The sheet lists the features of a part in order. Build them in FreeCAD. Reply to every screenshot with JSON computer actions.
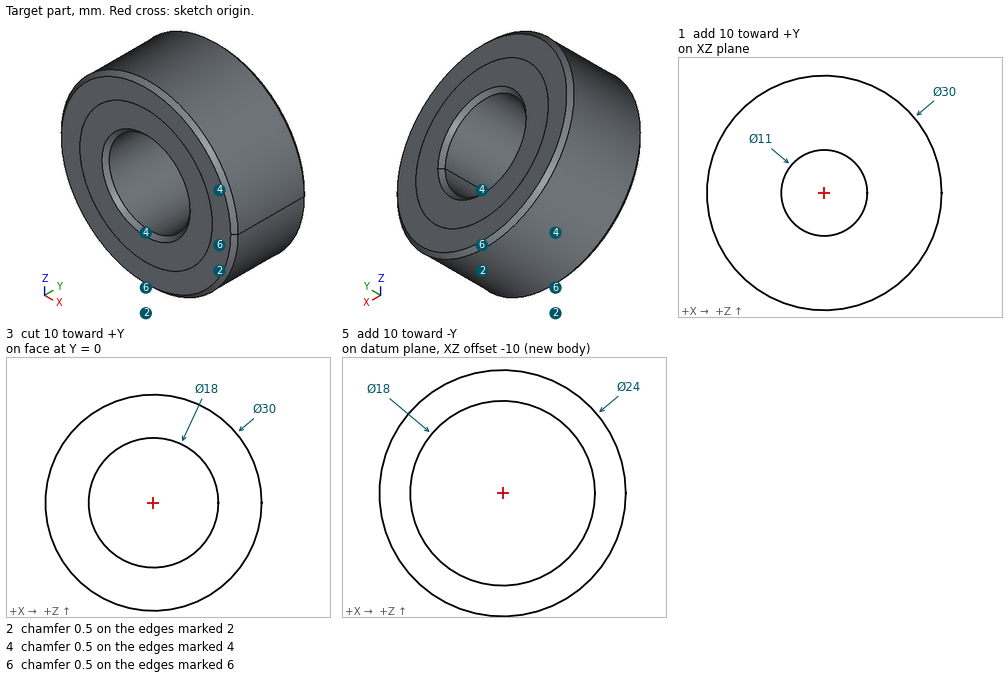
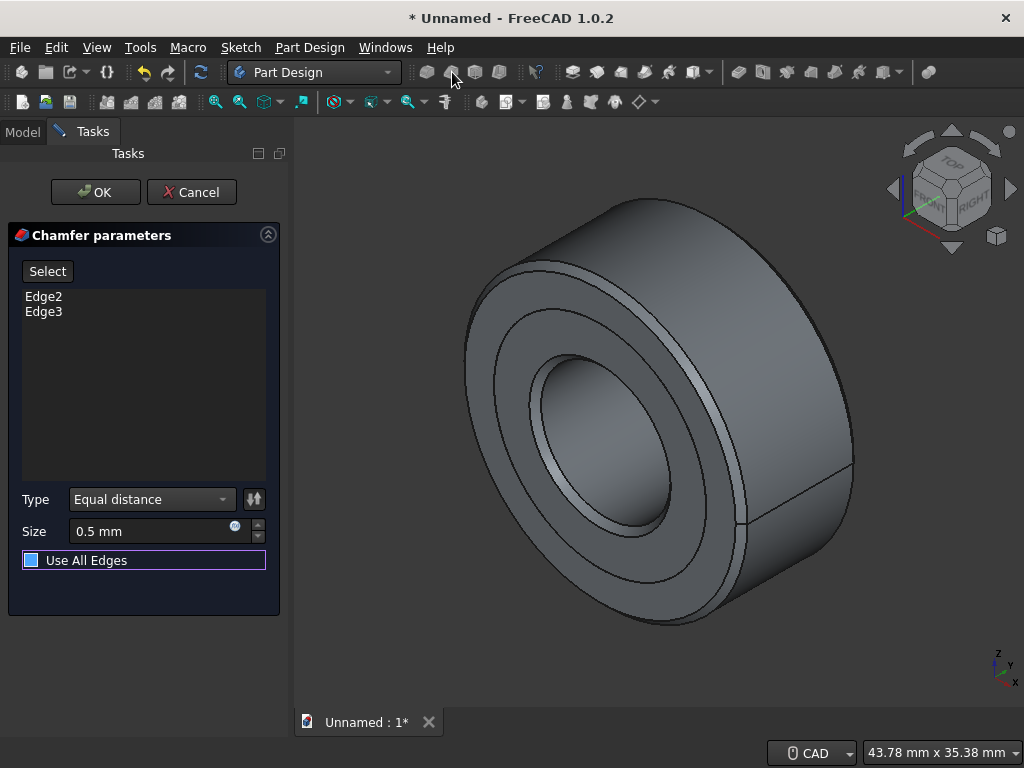
{"action": "left_click", "coordinate": [96, 192]}